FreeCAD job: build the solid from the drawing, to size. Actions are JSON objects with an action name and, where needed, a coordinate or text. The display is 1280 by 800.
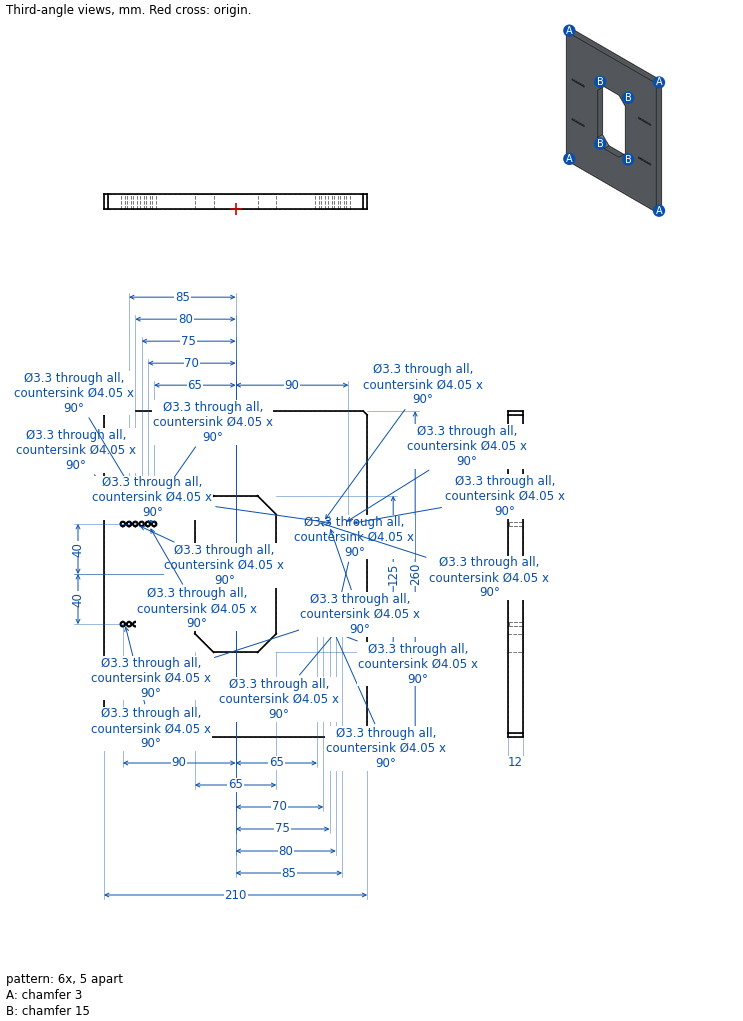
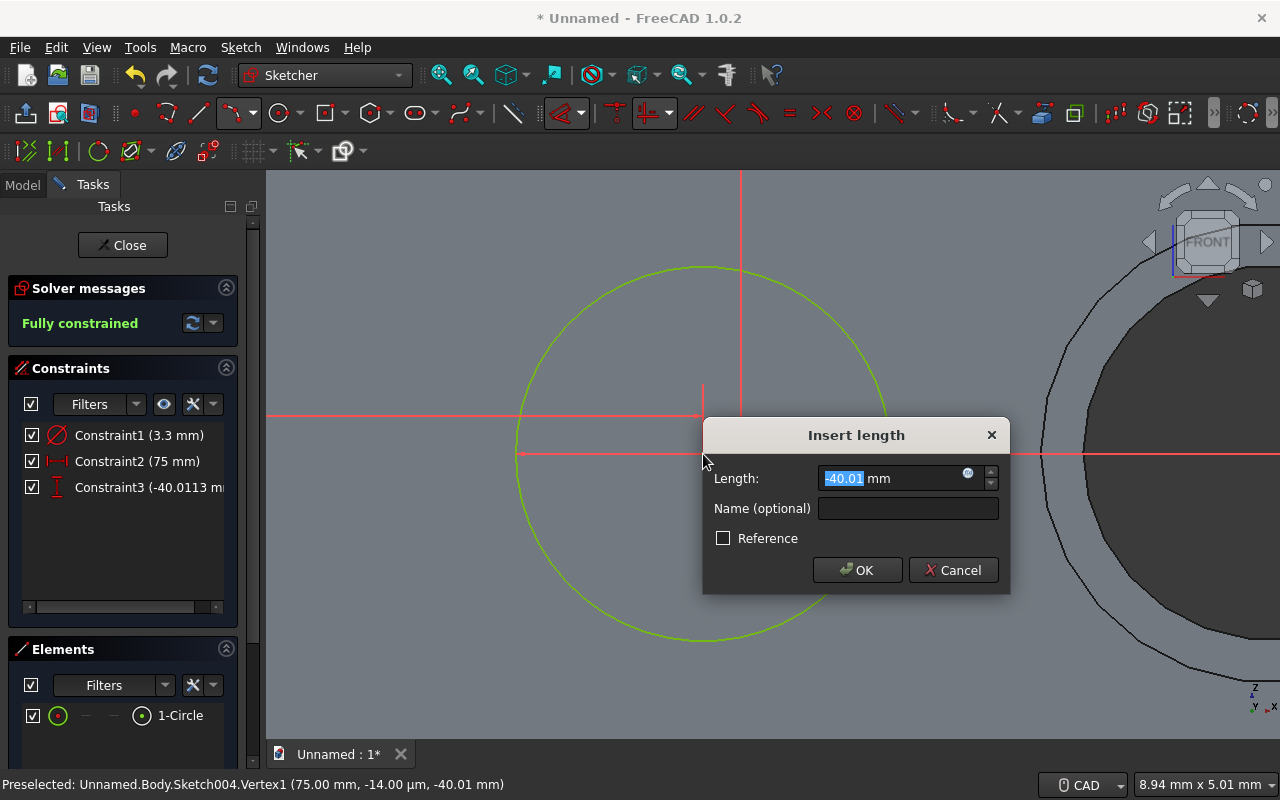
{"action": "type", "text": "-40"}
{"action": "key", "text": "Return"}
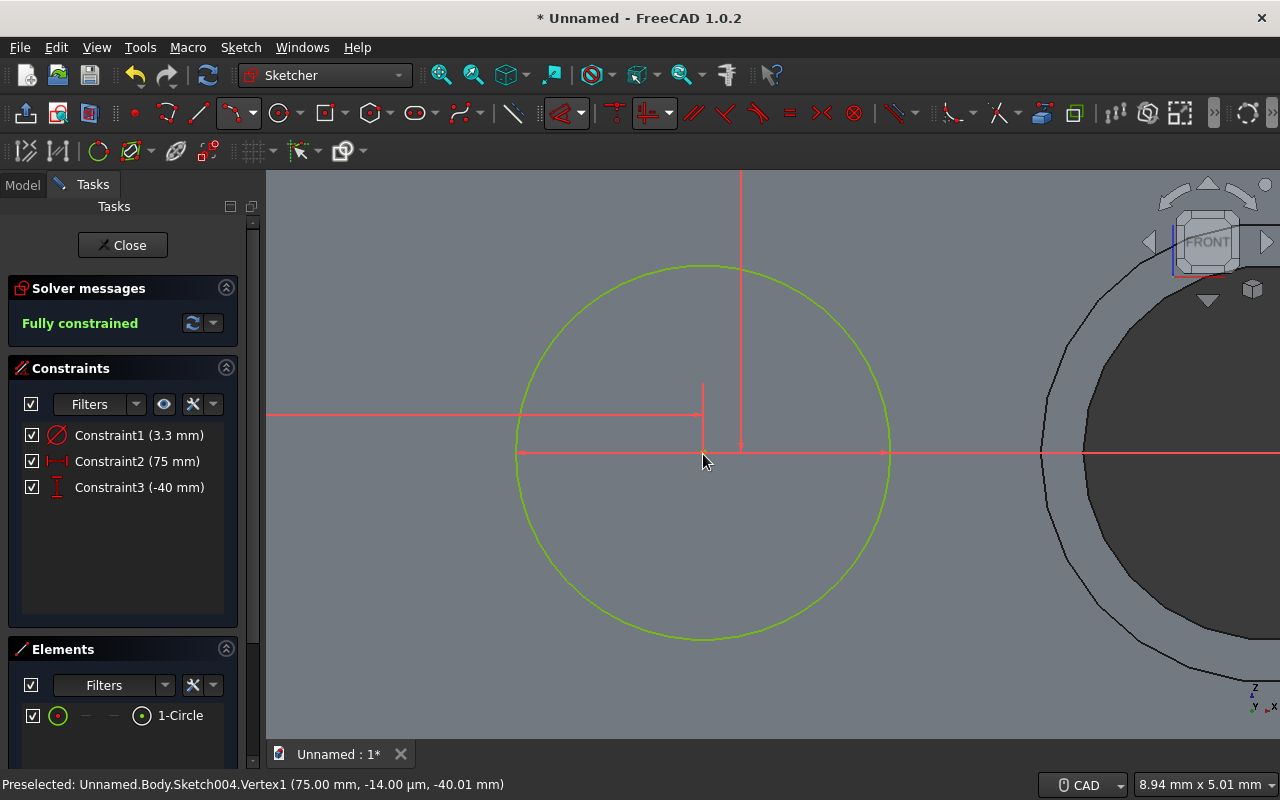
{"action": "left_click", "coordinate": [123, 245]}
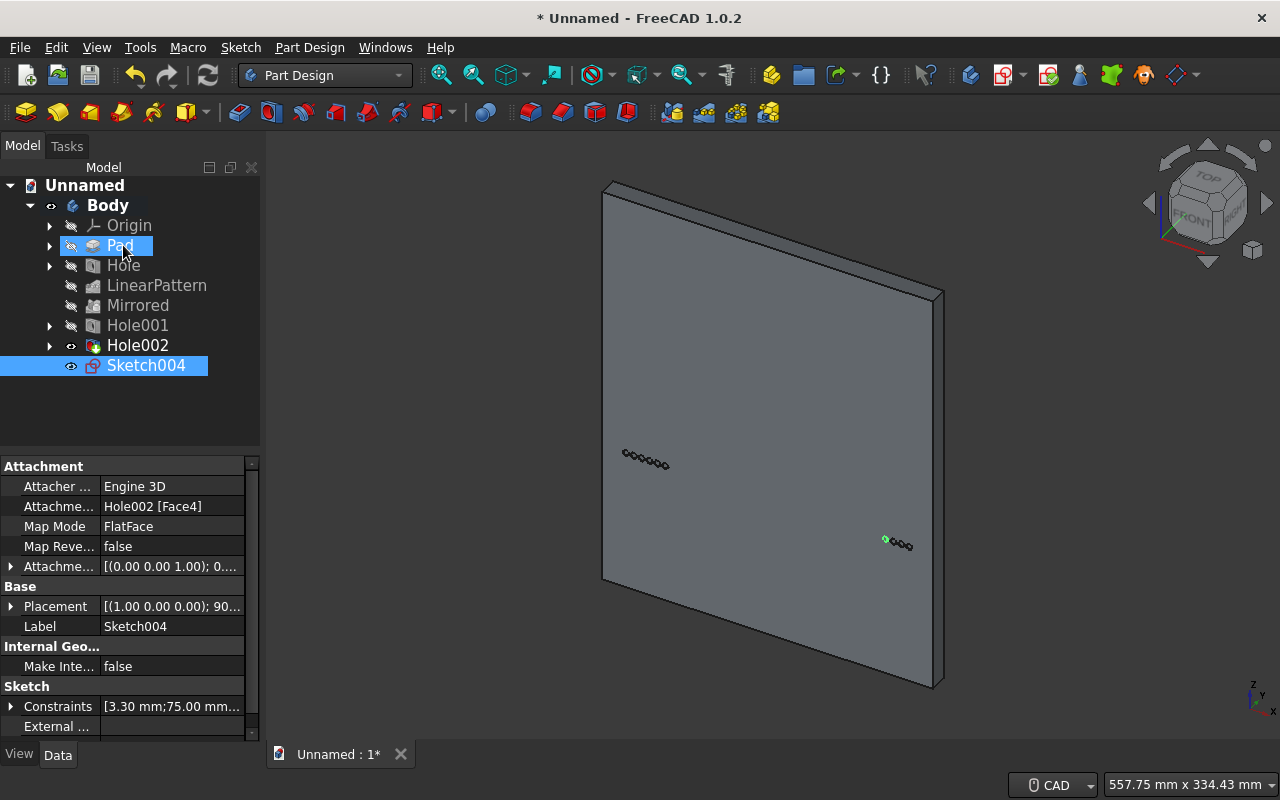
{"action": "left_click", "coordinate": [272, 112]}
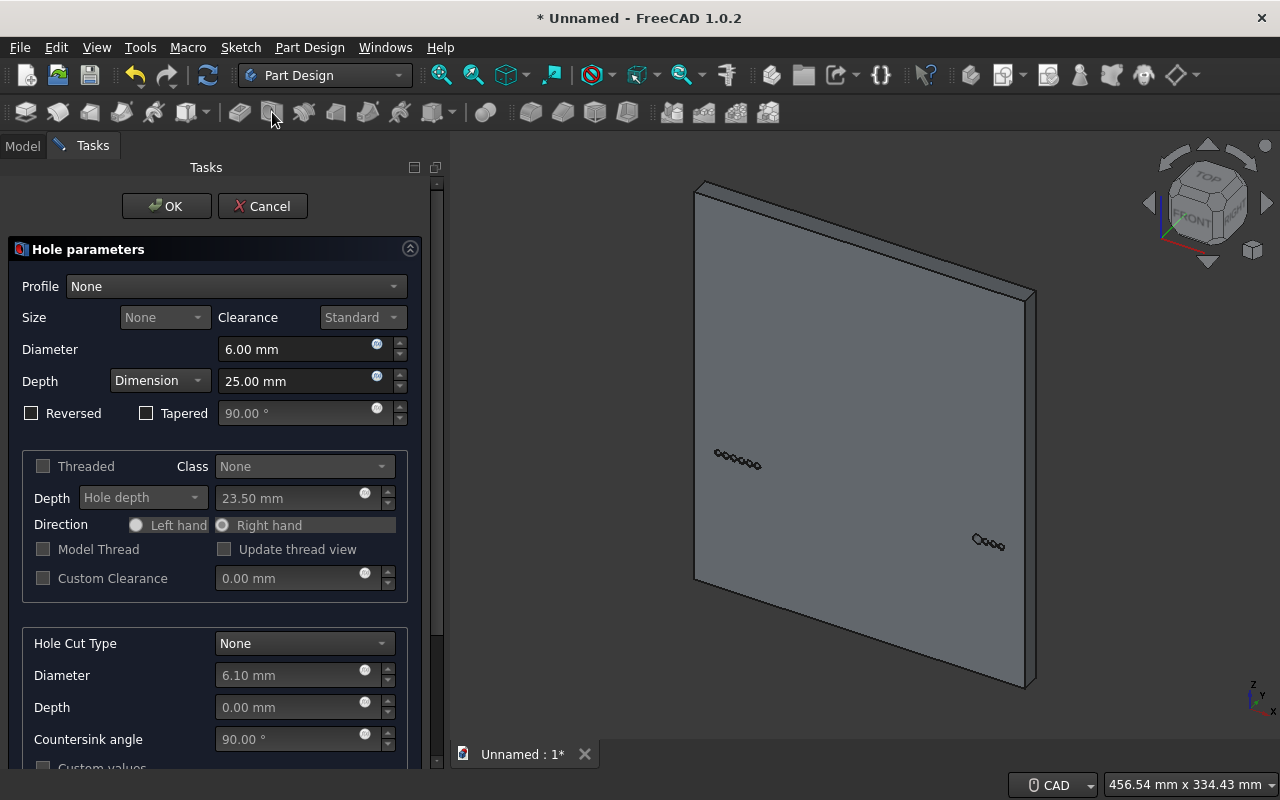
{"action": "triple_click", "coordinate": [305, 349]}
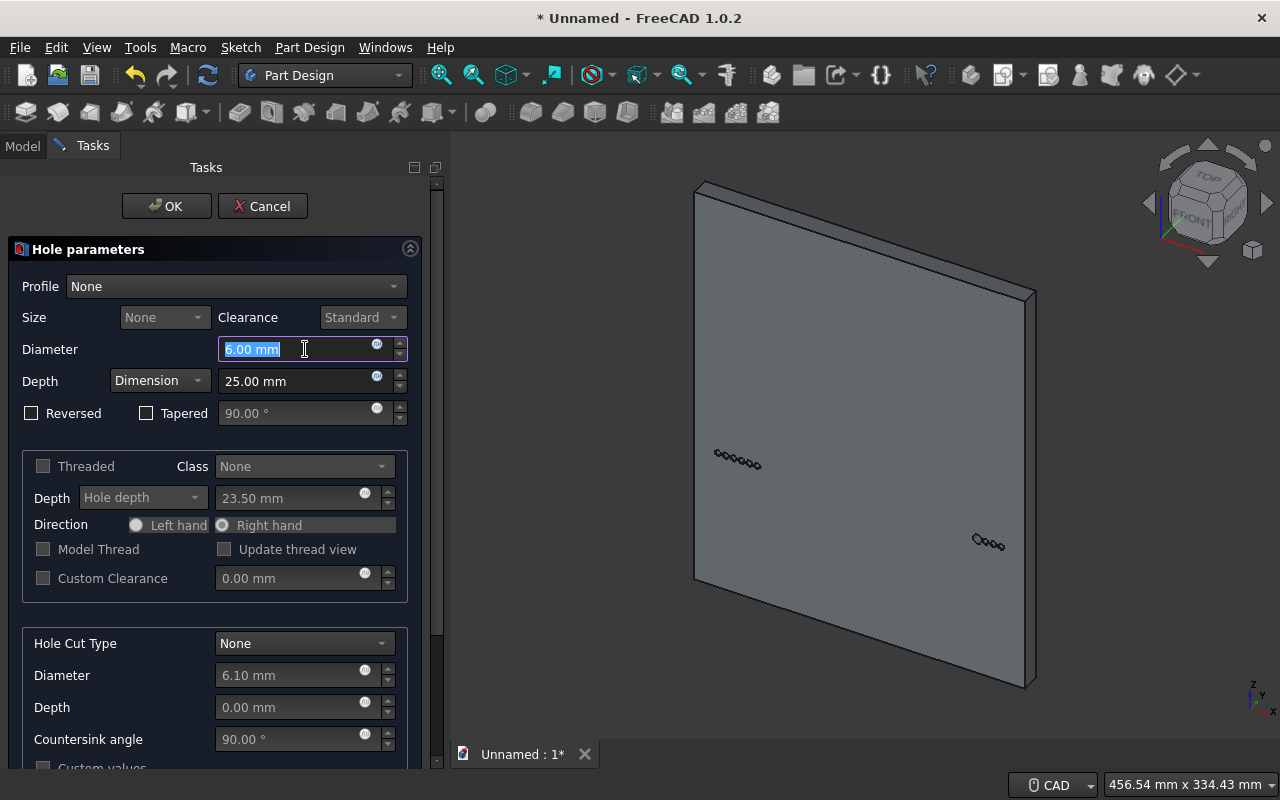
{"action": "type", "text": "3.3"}
{"action": "key", "text": "Tab"}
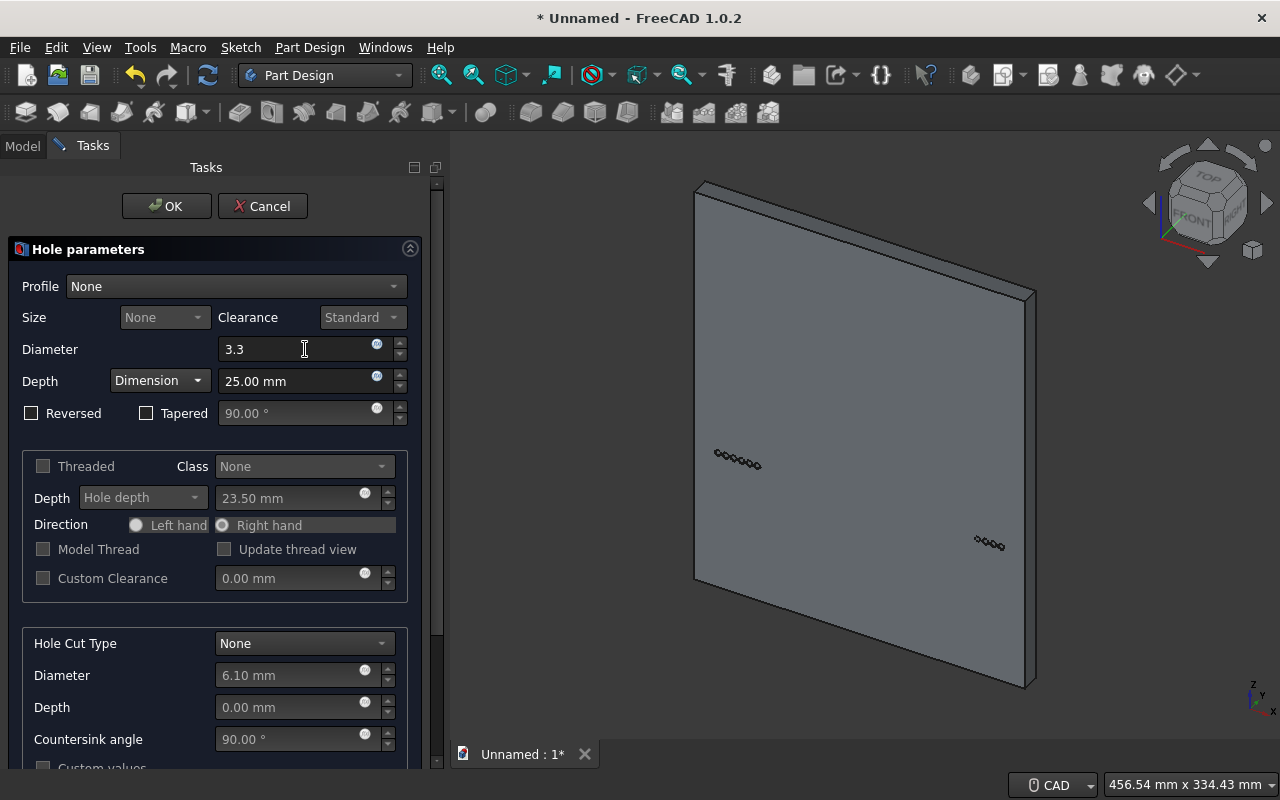
{"action": "left_click", "coordinate": [161, 380]}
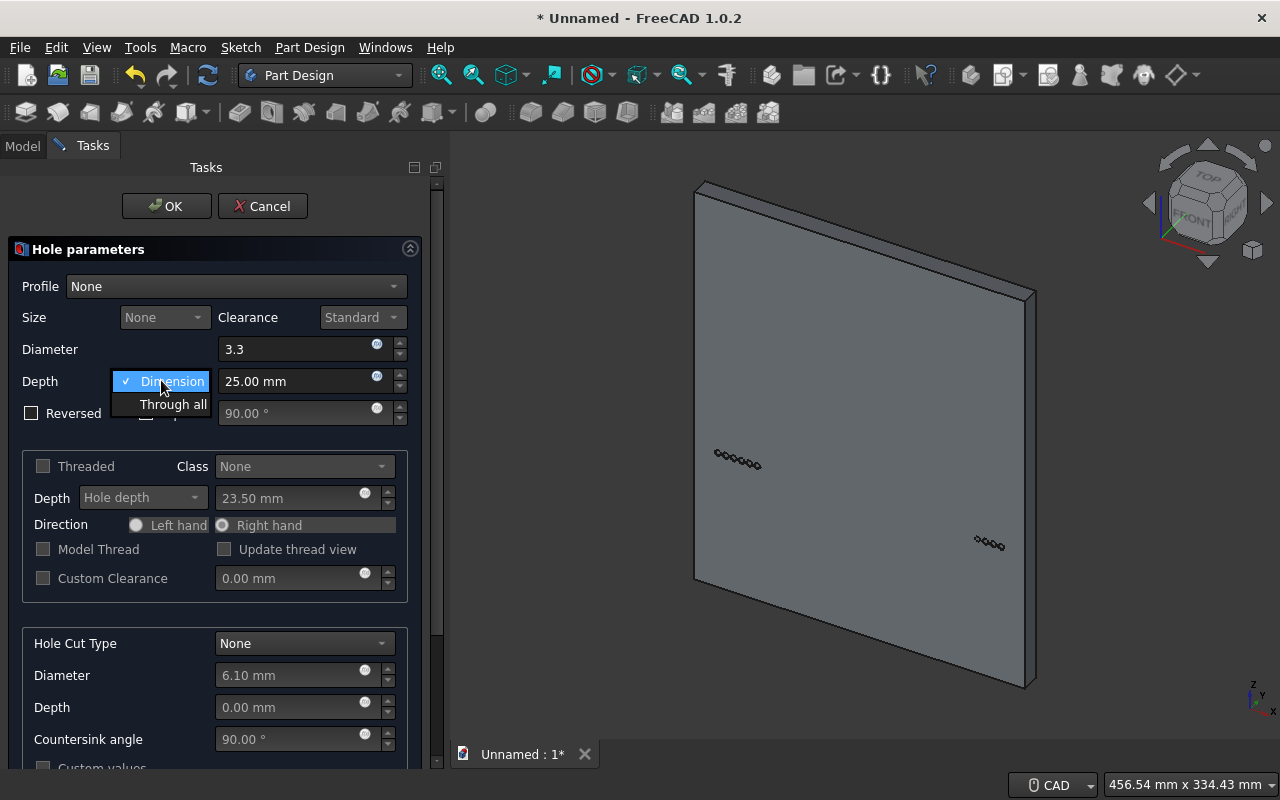
{"action": "left_click", "coordinate": [160, 404]}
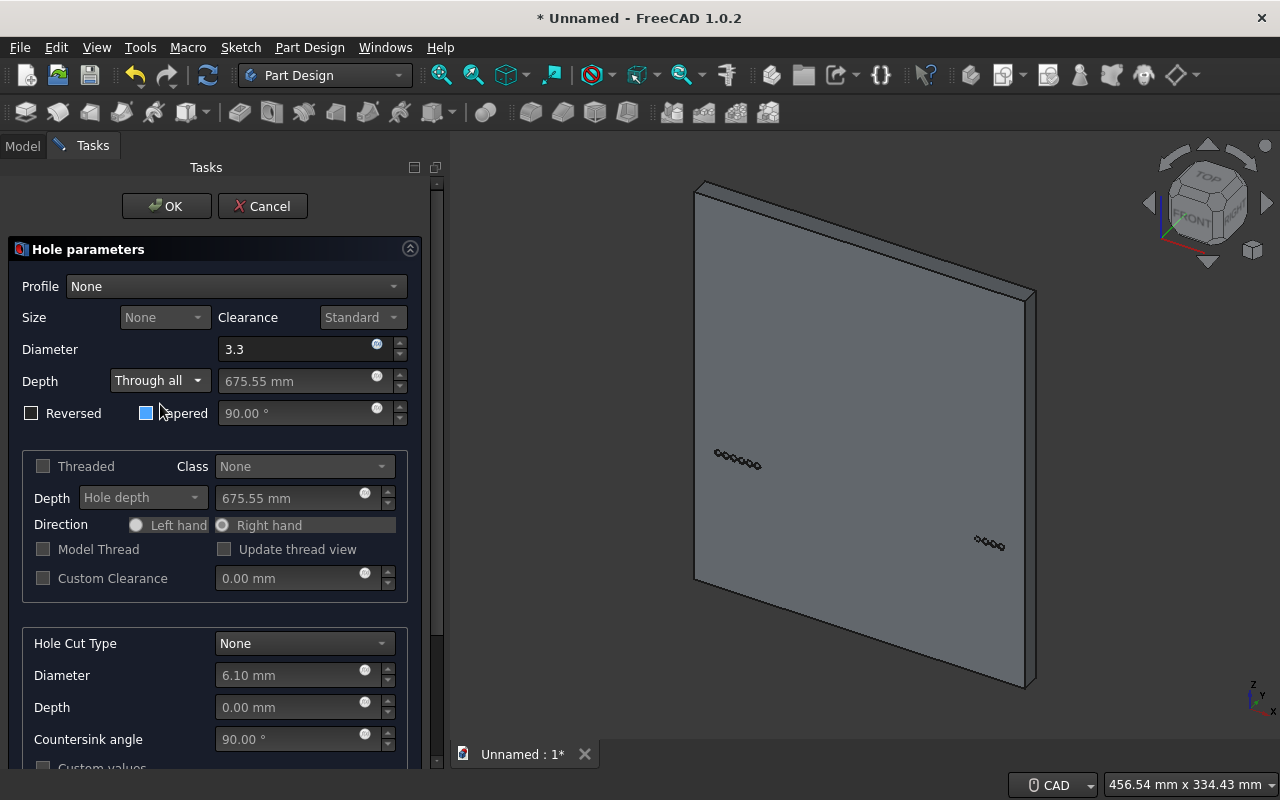
{"action": "left_click", "coordinate": [306, 644]}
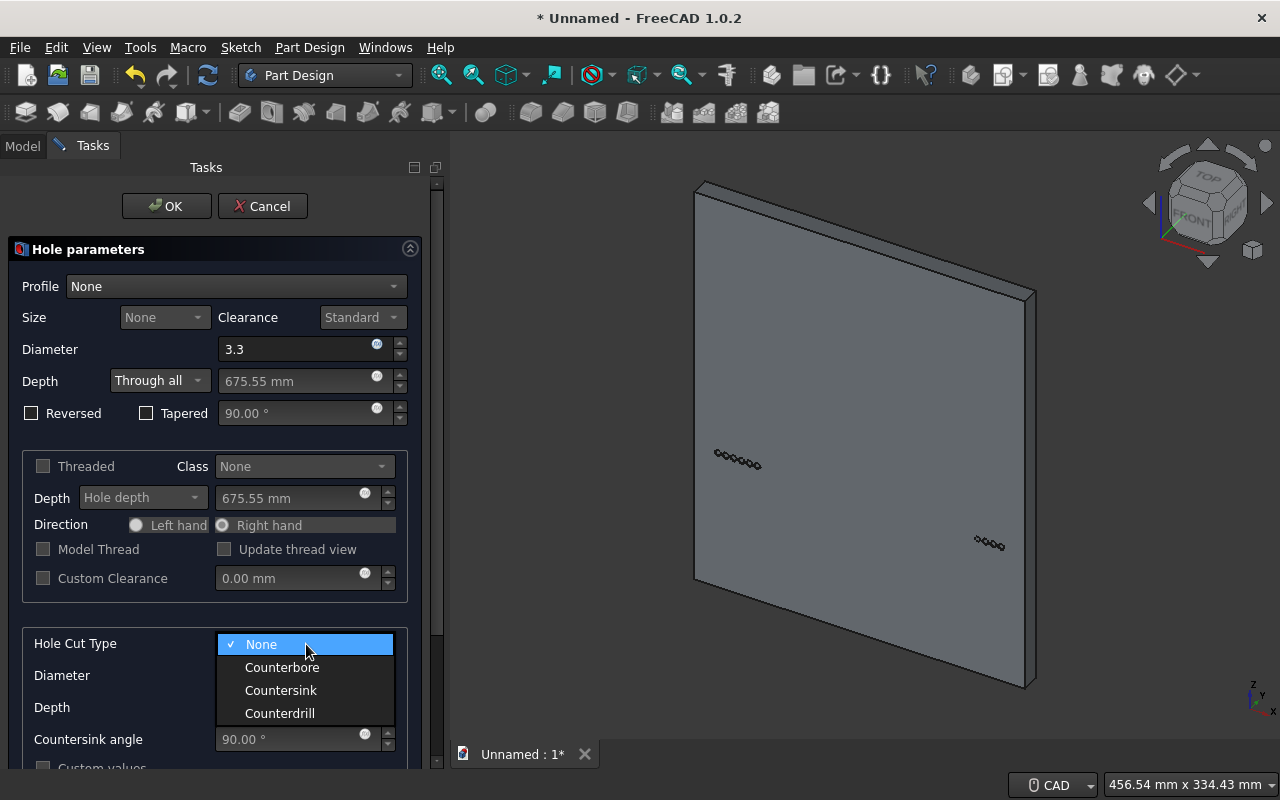
{"action": "left_click", "coordinate": [304, 690]}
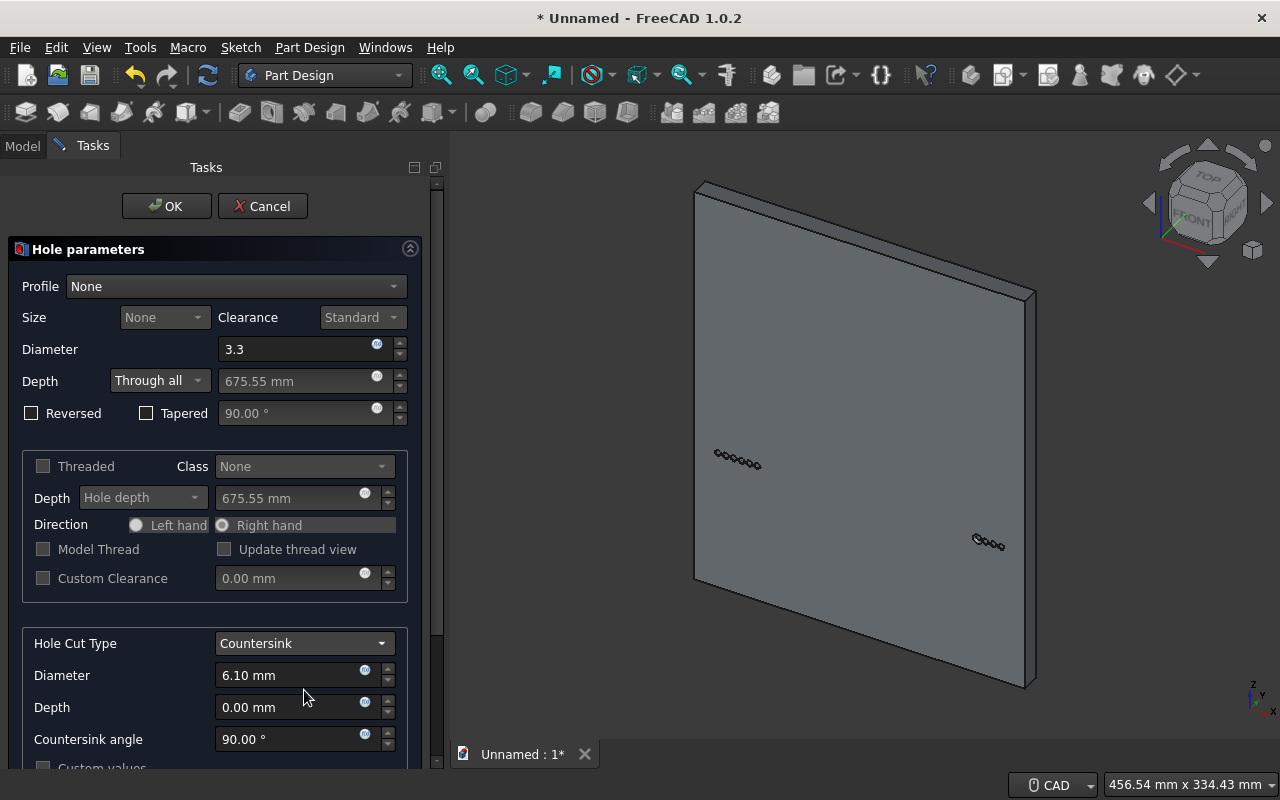
{"action": "triple_click", "coordinate": [298, 675]}